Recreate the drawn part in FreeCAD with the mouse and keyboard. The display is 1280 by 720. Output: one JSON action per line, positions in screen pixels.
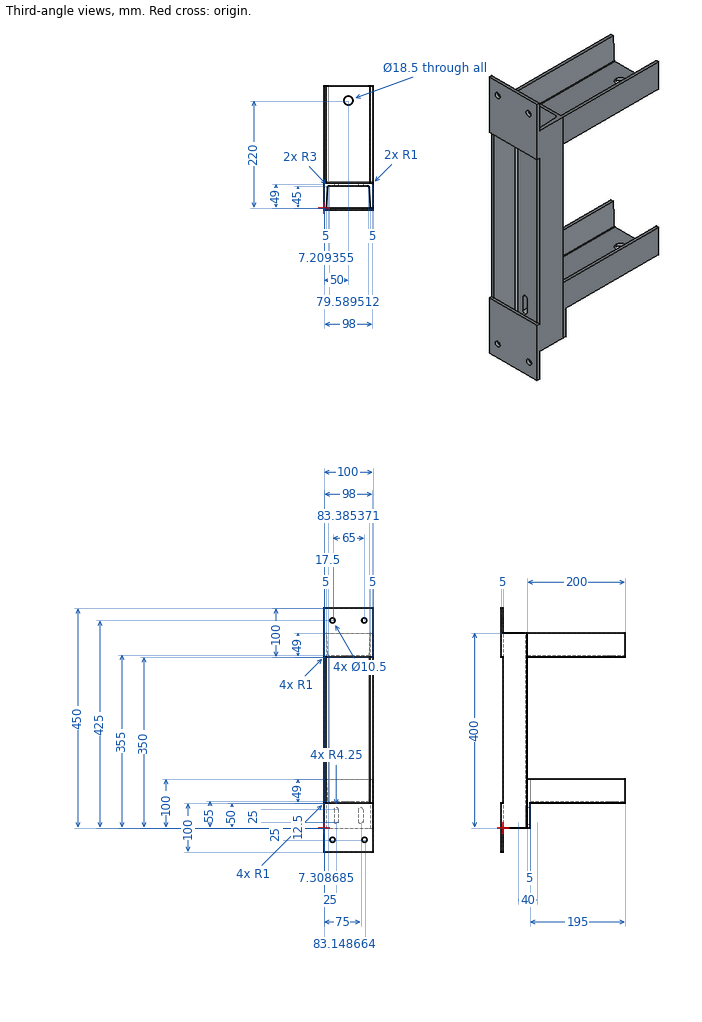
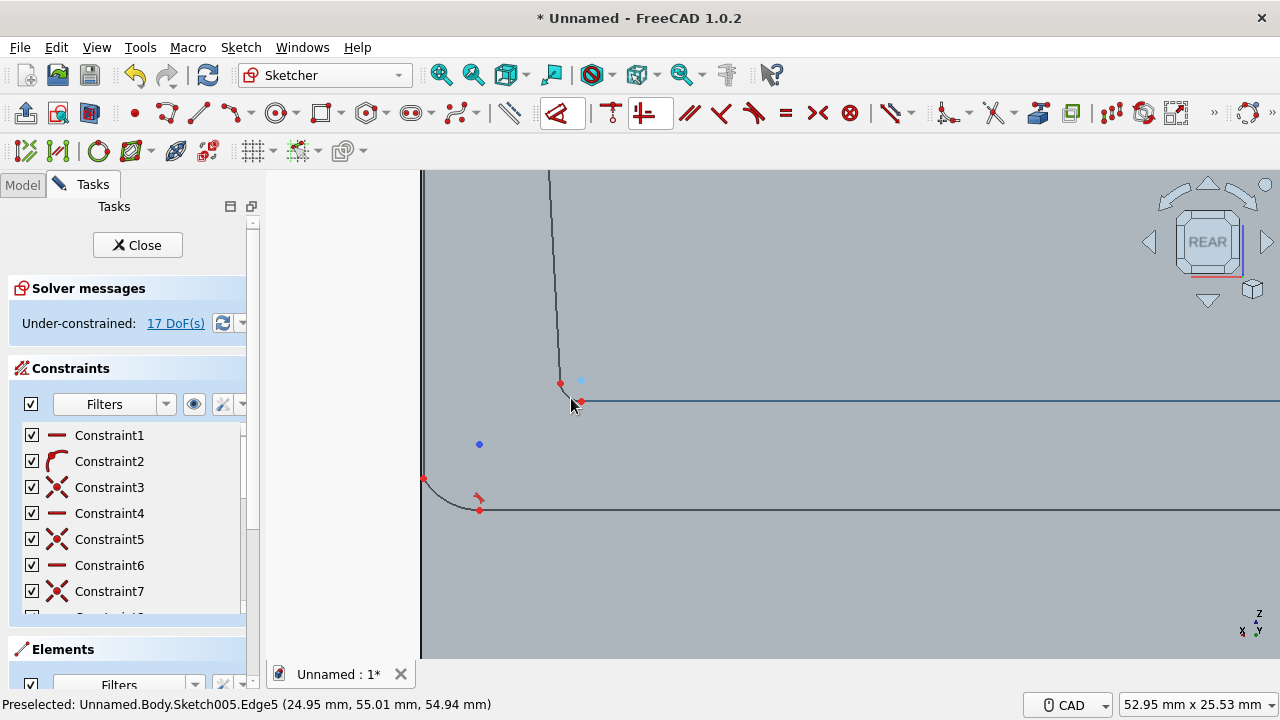
{"action": "left_click", "coordinate": [568, 396]}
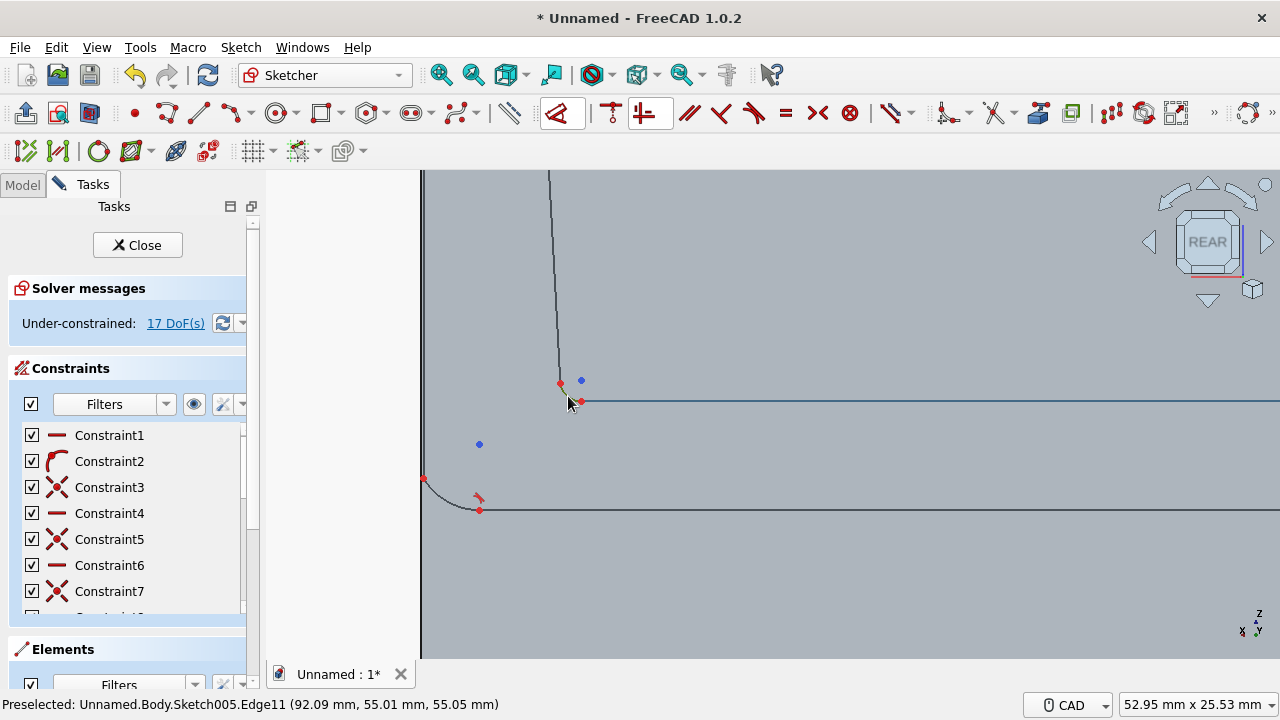
{"action": "key", "text": "t"}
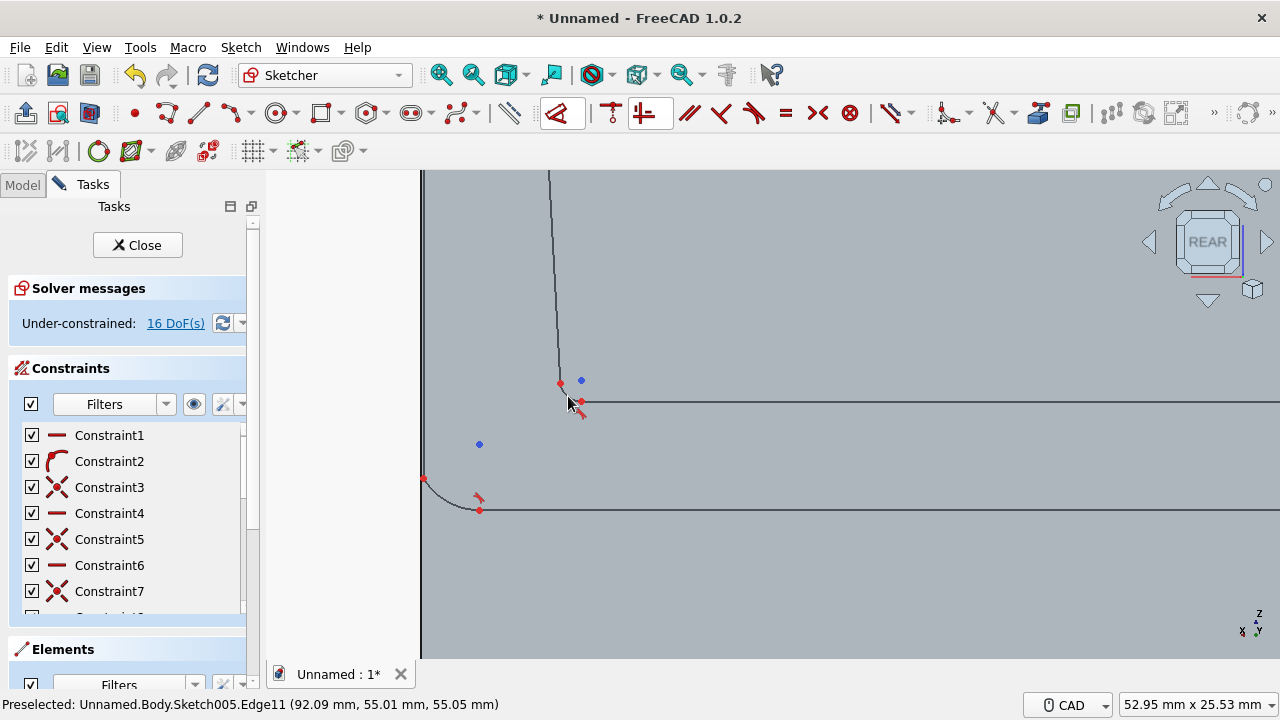
{"action": "scroll", "coordinate": [571, 398], "scroll_direction": "down", "scroll_amount": 9}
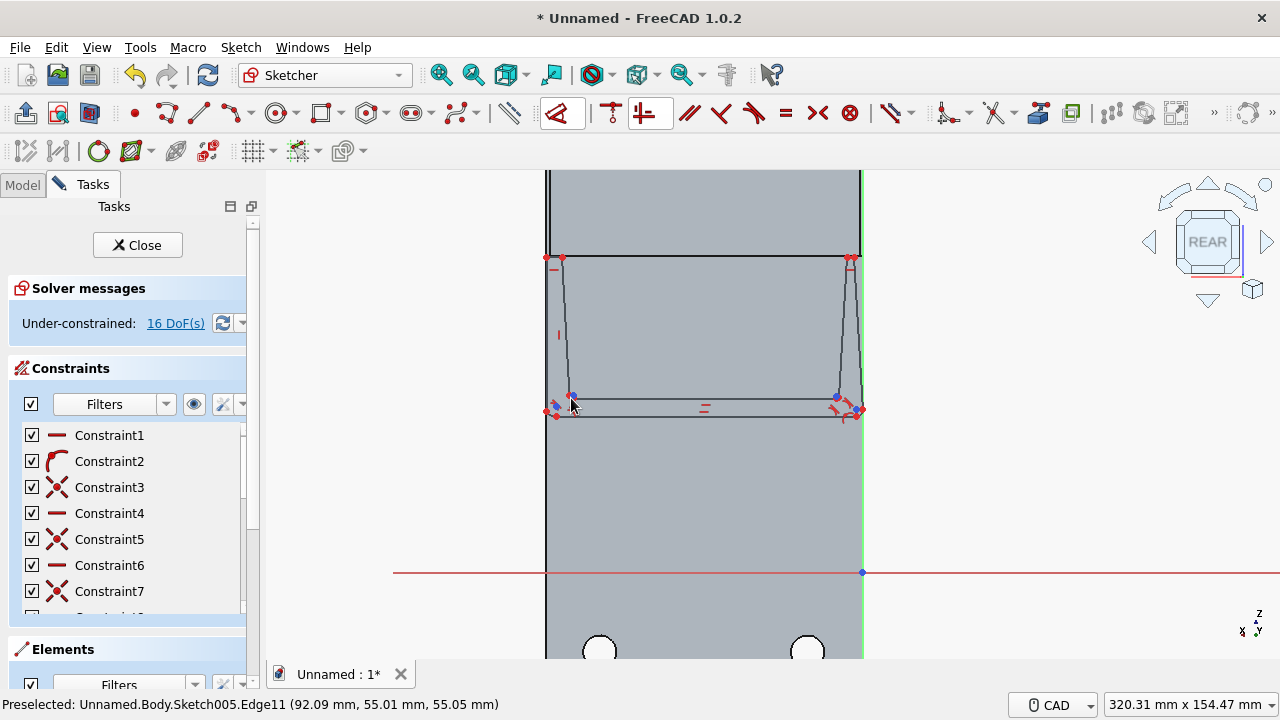
{"action": "left_click", "coordinate": [568, 368]}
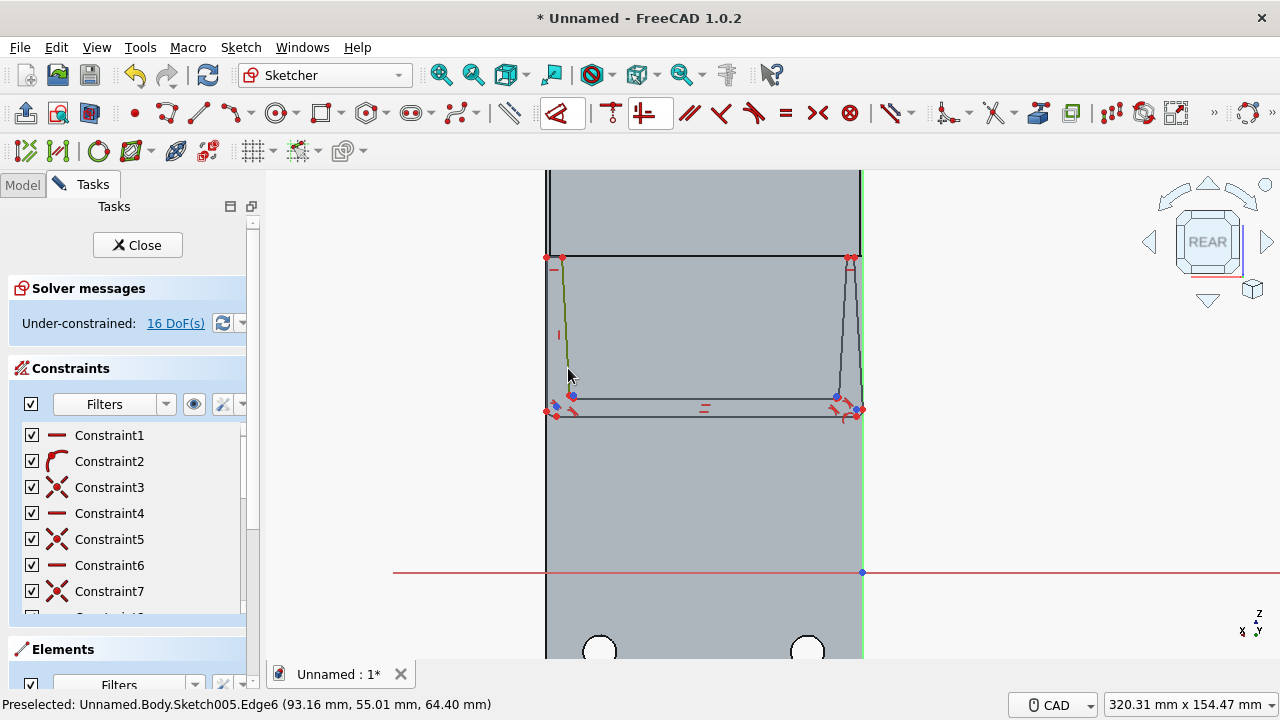
{"action": "scroll", "coordinate": [571, 398], "scroll_direction": "up", "scroll_amount": 9}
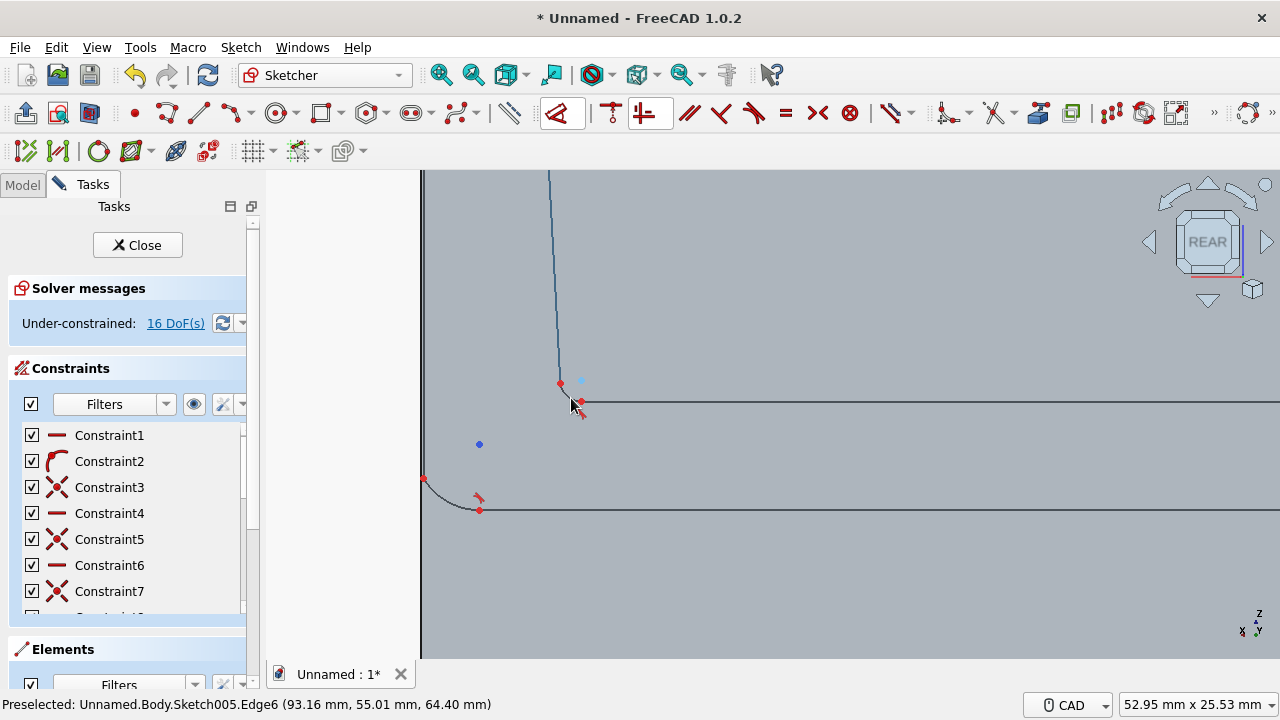
{"action": "left_click", "coordinate": [568, 396]}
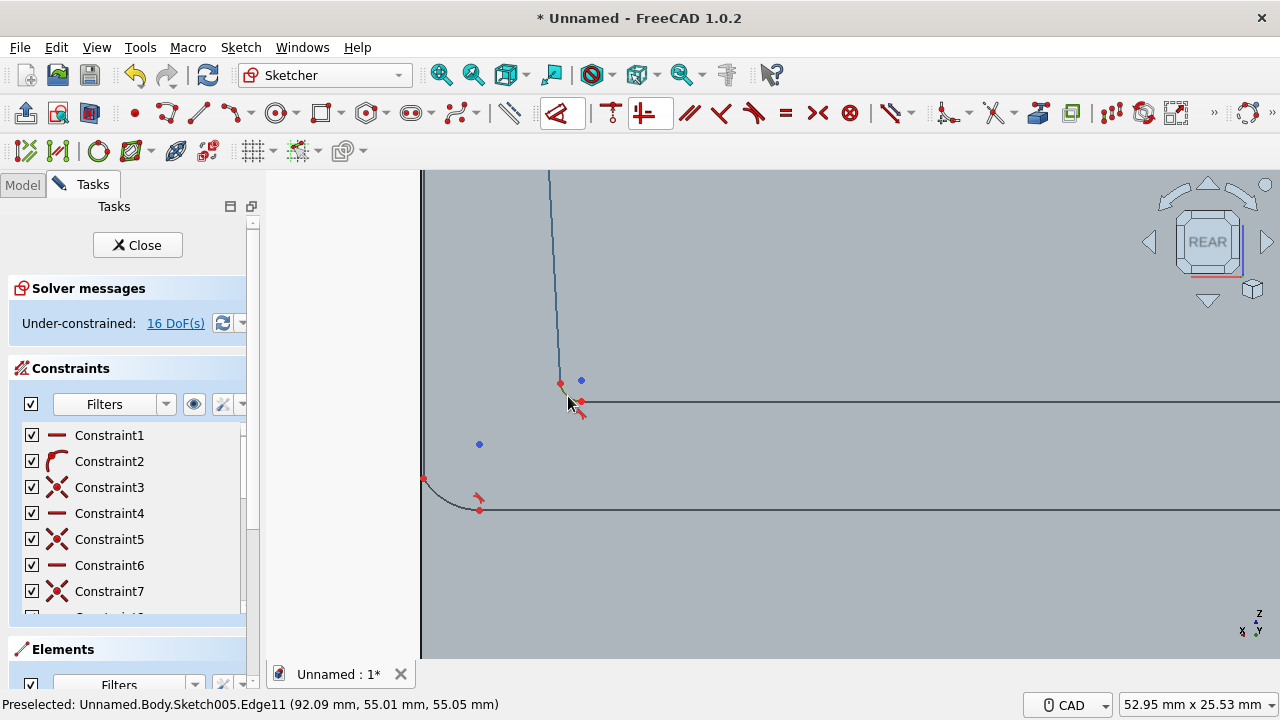
{"action": "left_click", "coordinate": [754, 114]}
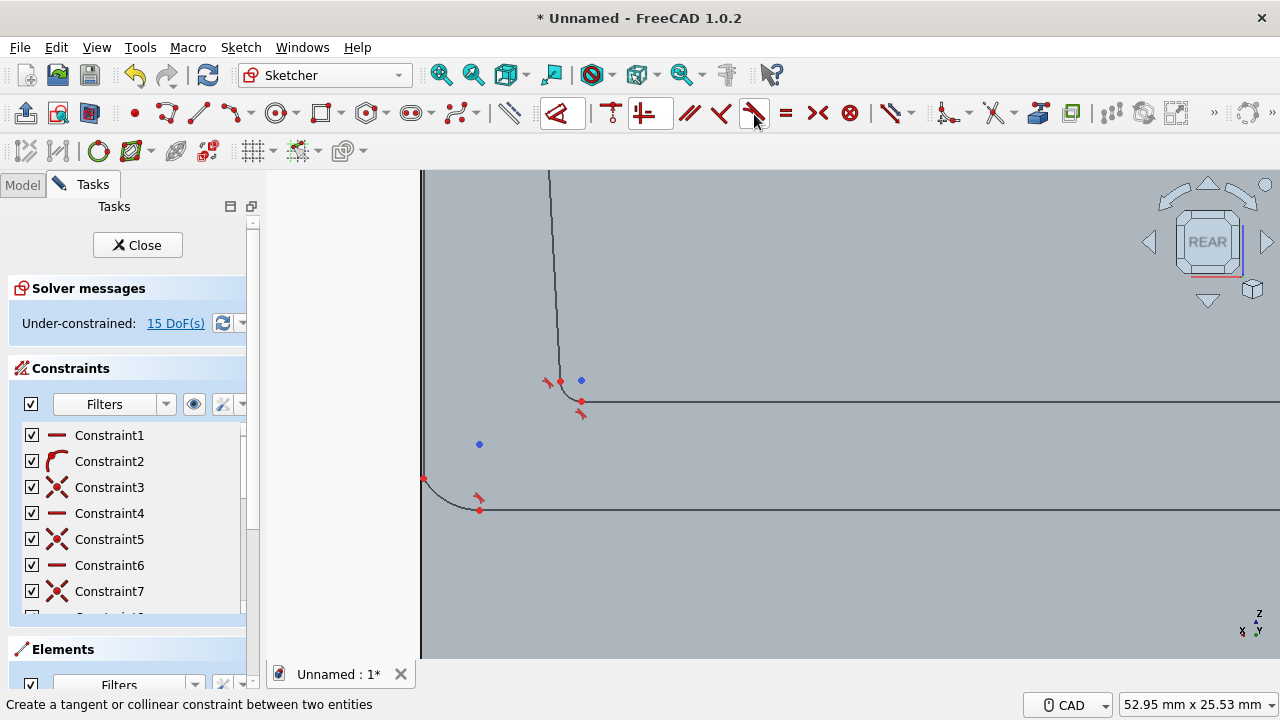
{"action": "scroll", "coordinate": [571, 398], "scroll_direction": "down", "scroll_amount": 9}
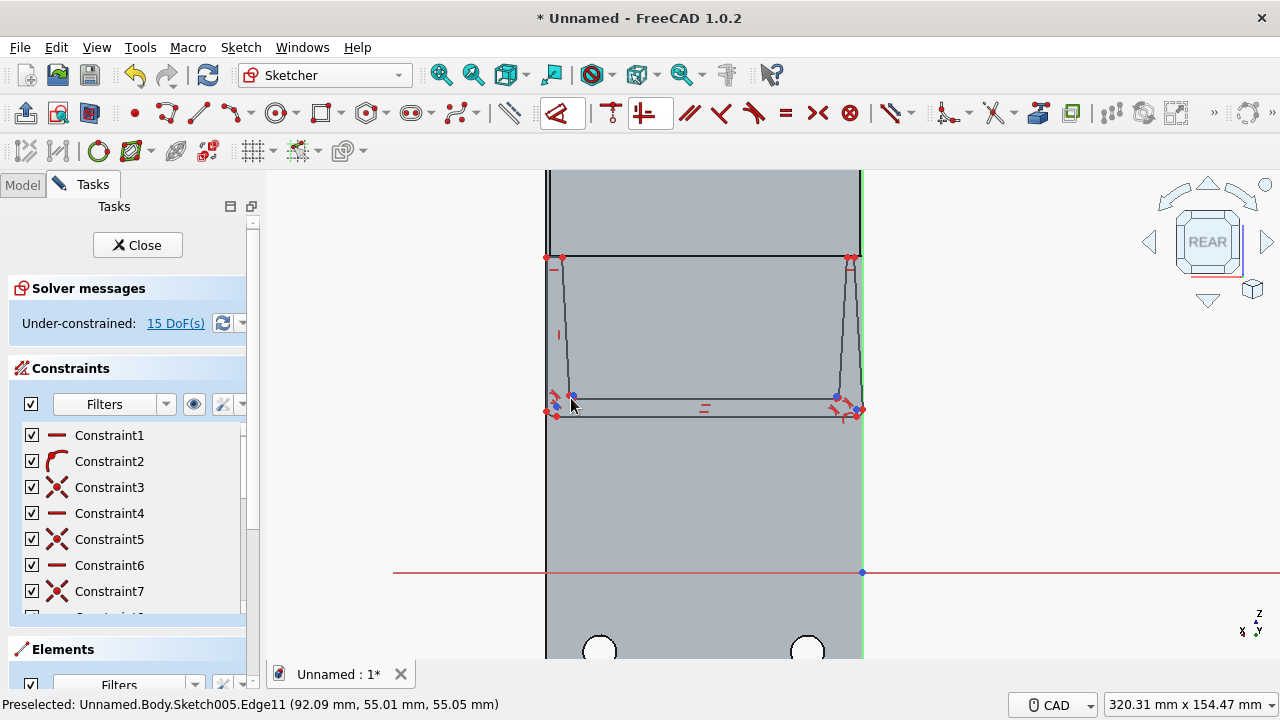
{"action": "left_click", "coordinate": [547, 365]}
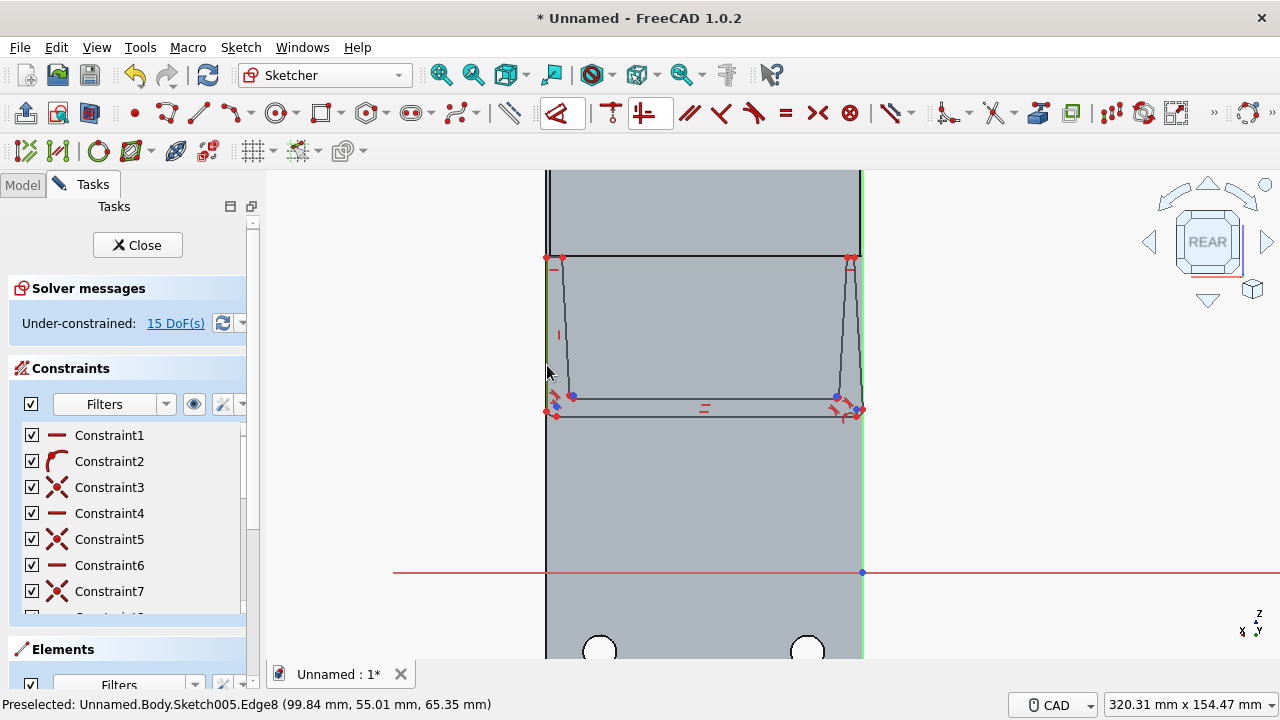
{"action": "scroll", "coordinate": [551, 416], "scroll_direction": "up", "scroll_amount": 5}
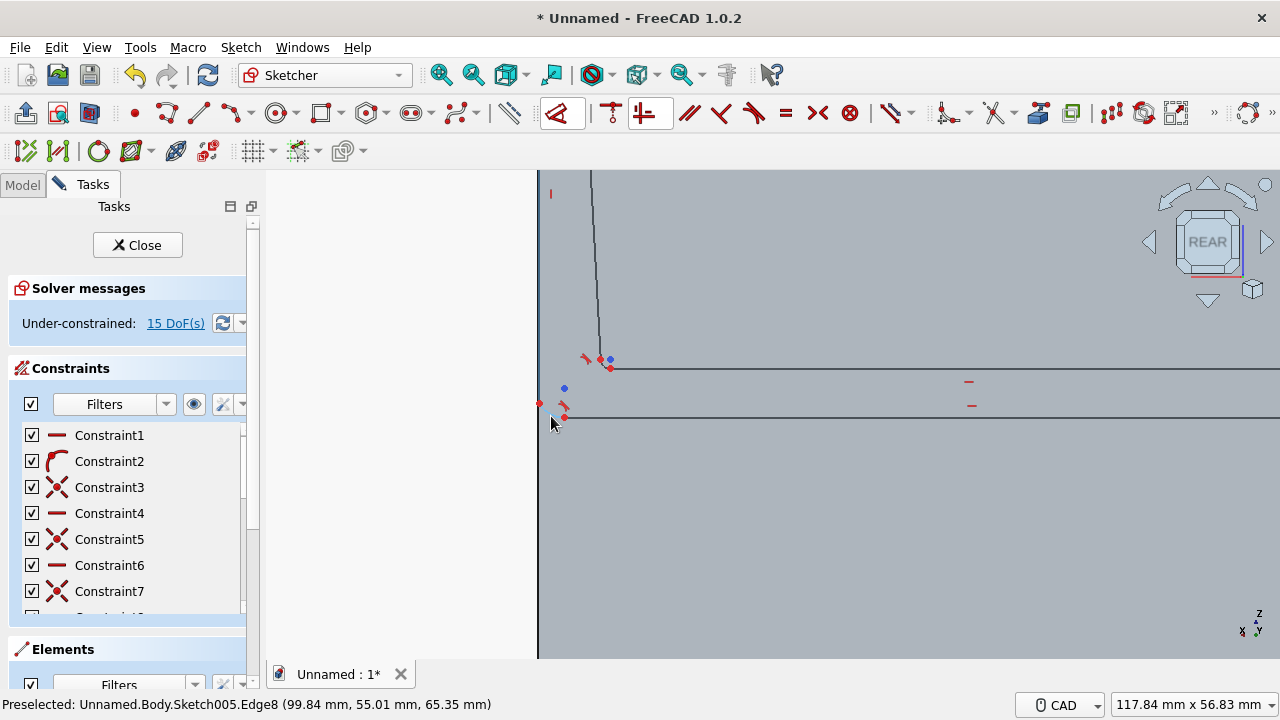
{"action": "left_click", "coordinate": [550, 414]}